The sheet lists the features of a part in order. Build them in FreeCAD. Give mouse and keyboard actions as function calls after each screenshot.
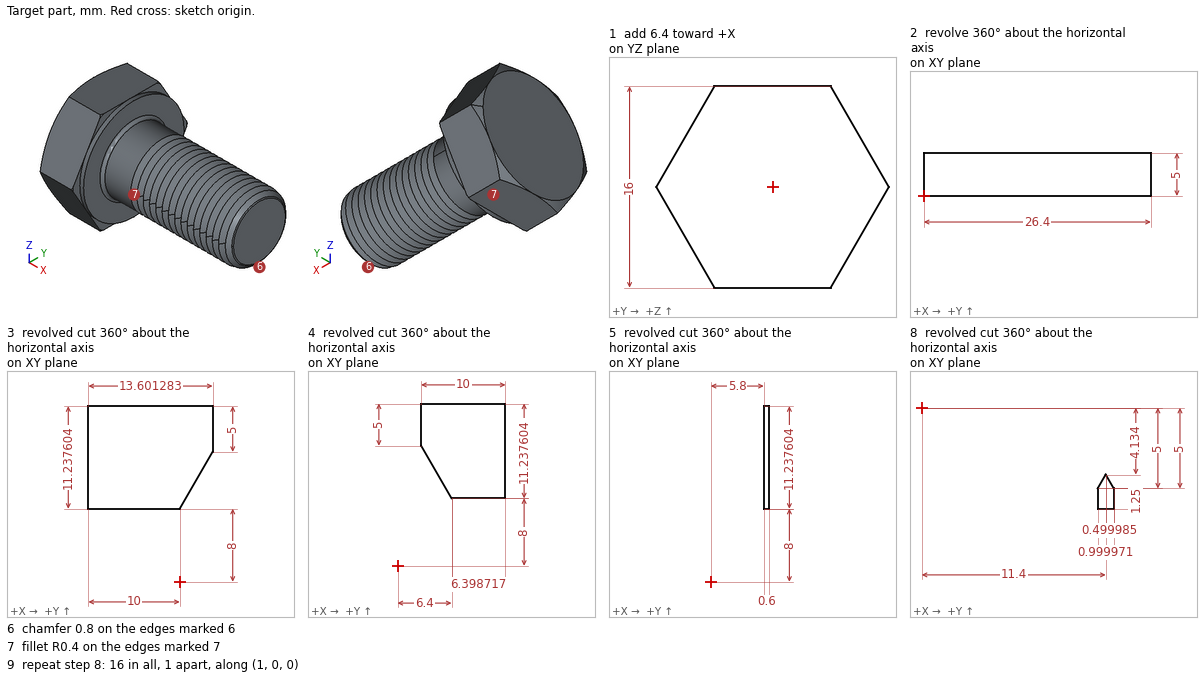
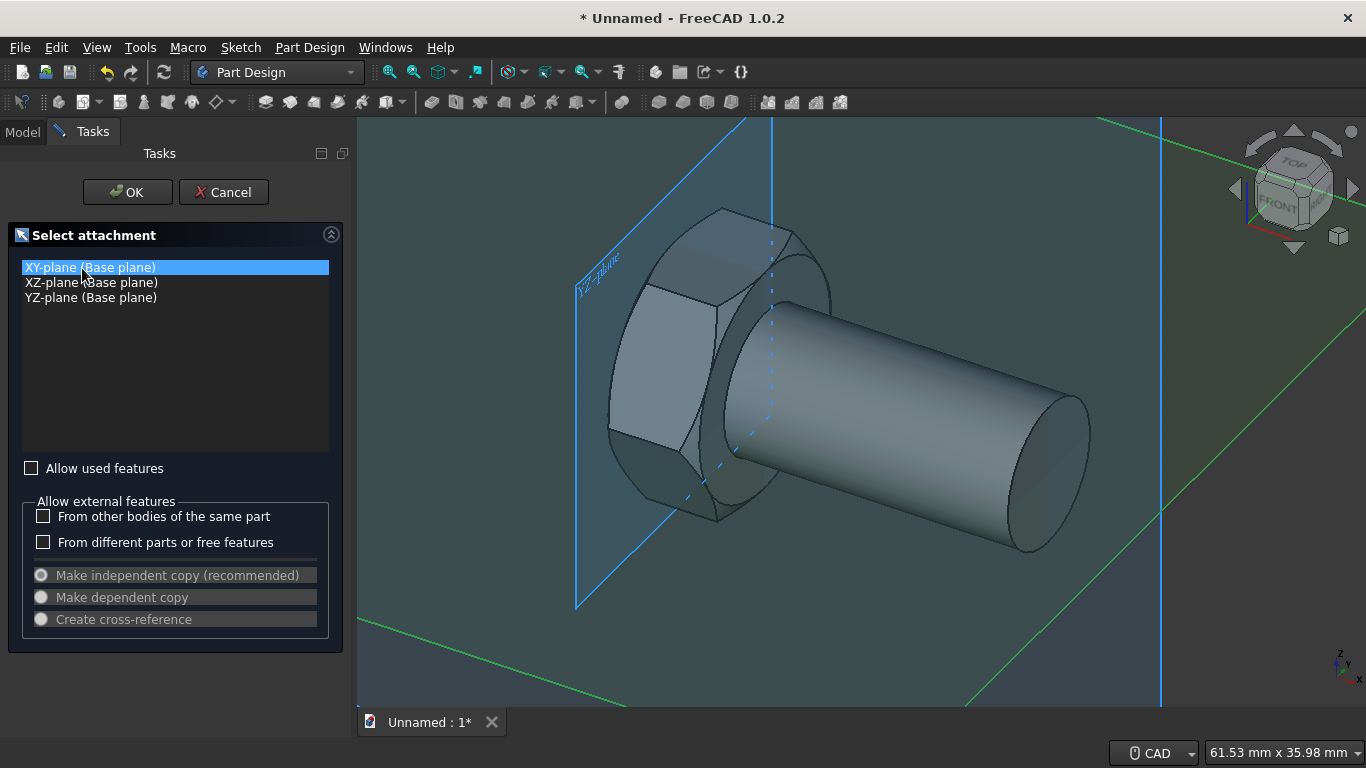
click(128, 192)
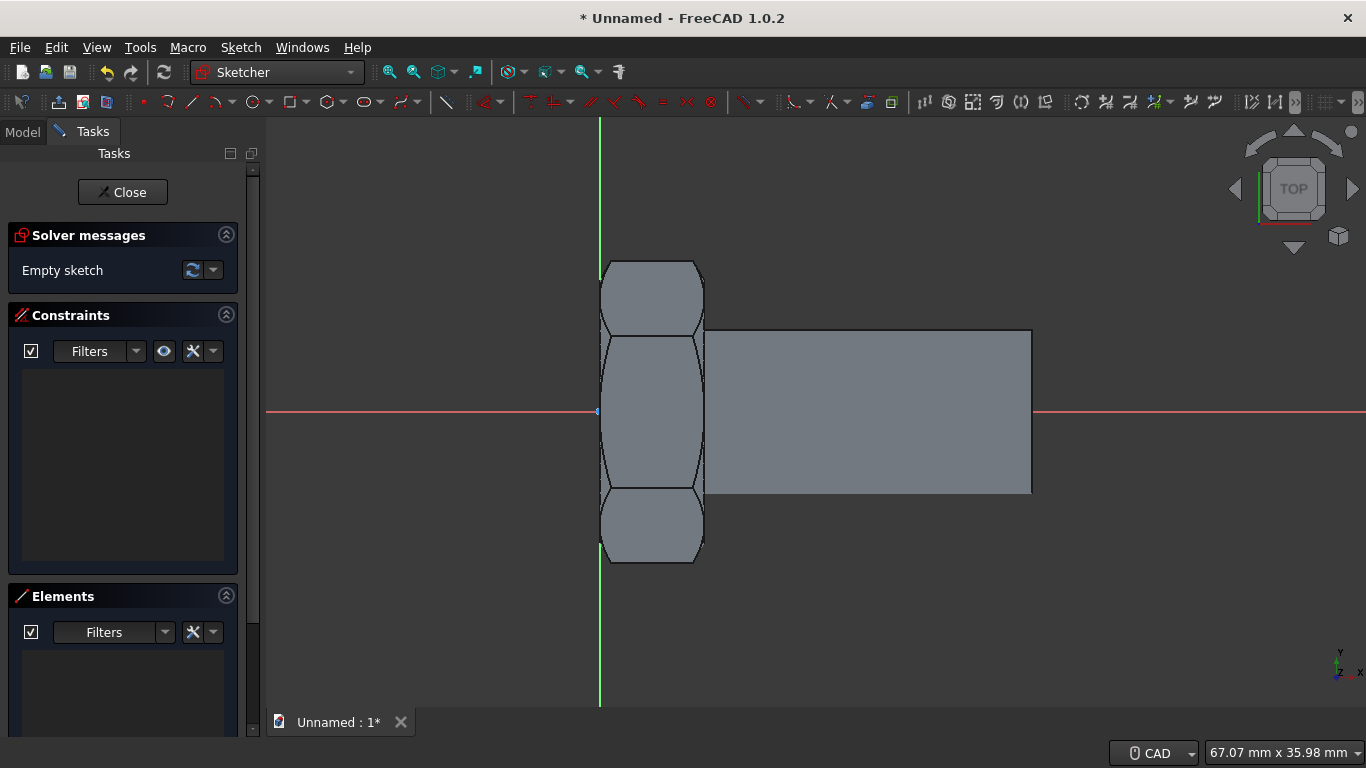
click(108, 102)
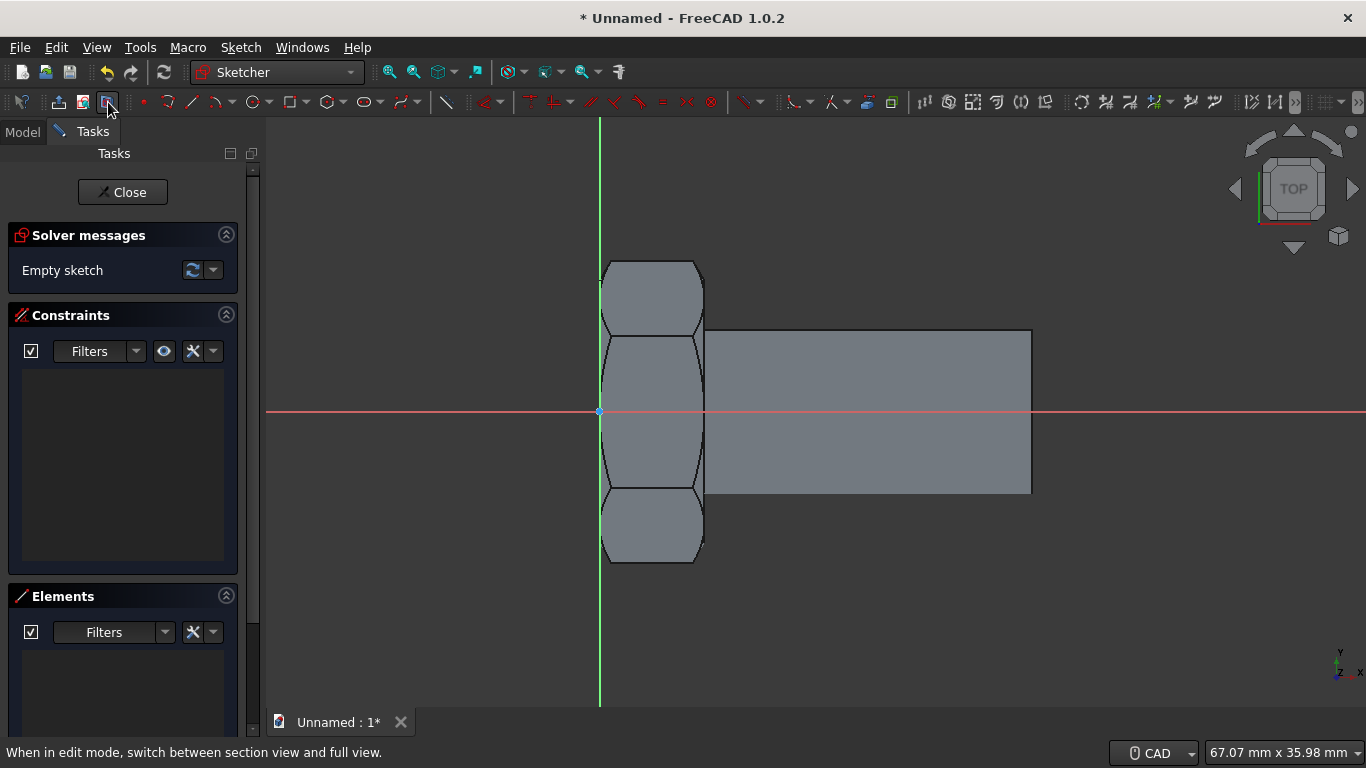
scroll(1179, 679, down, 1)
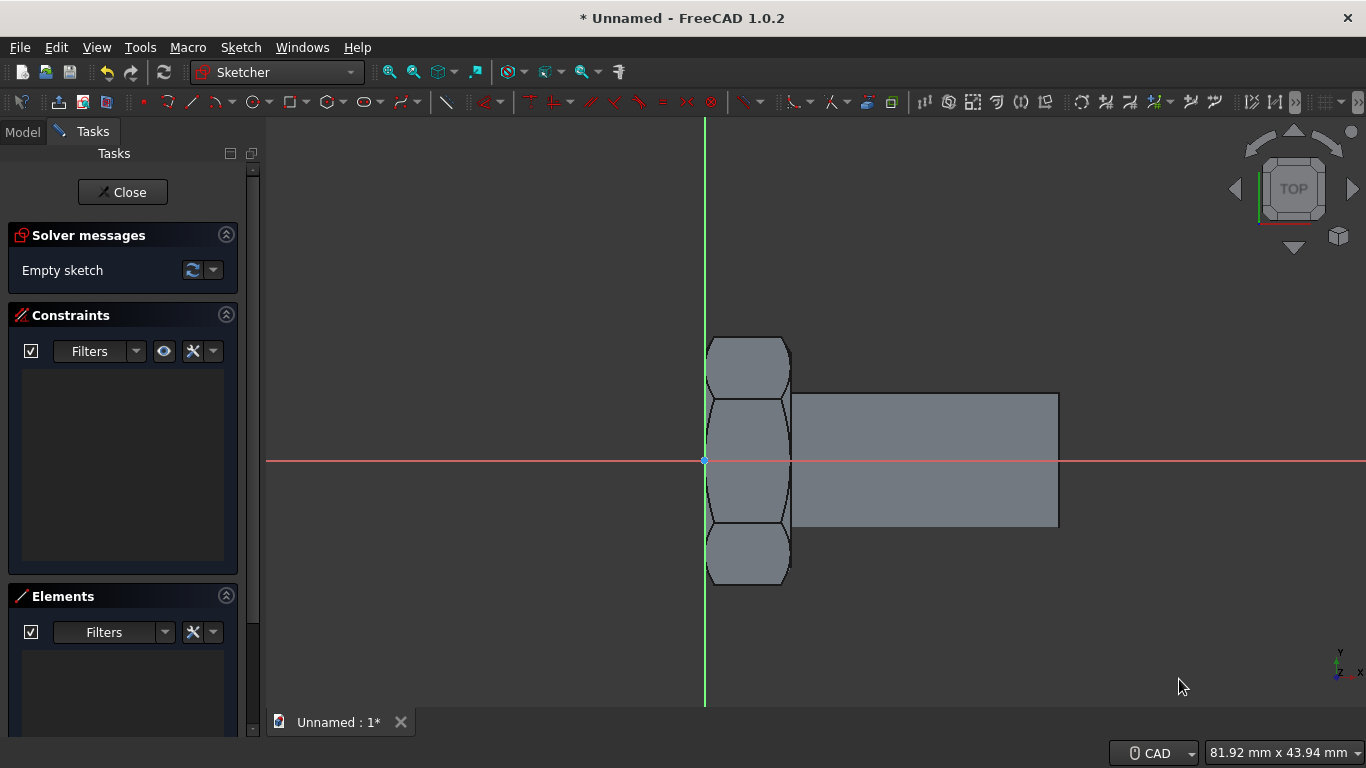
scroll(748, 168, up, 2)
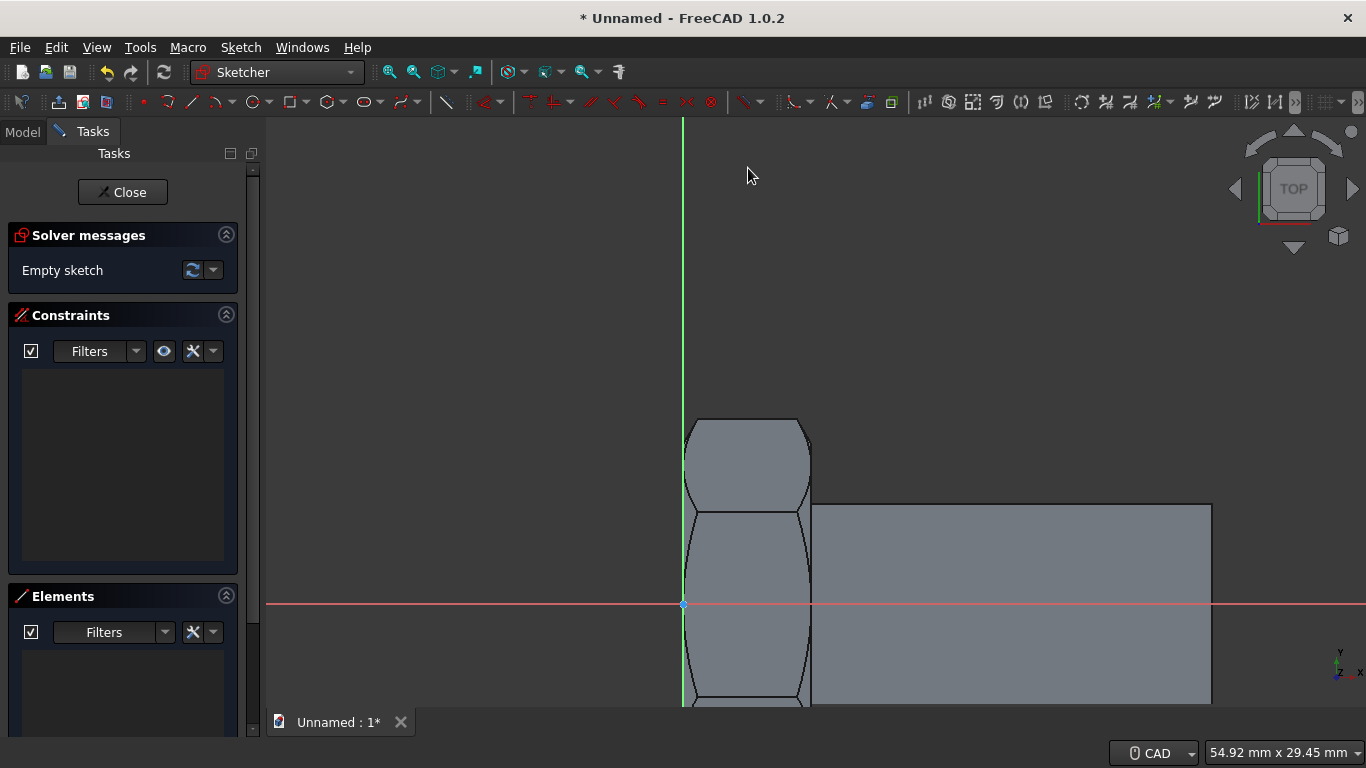
key(g)
key(r)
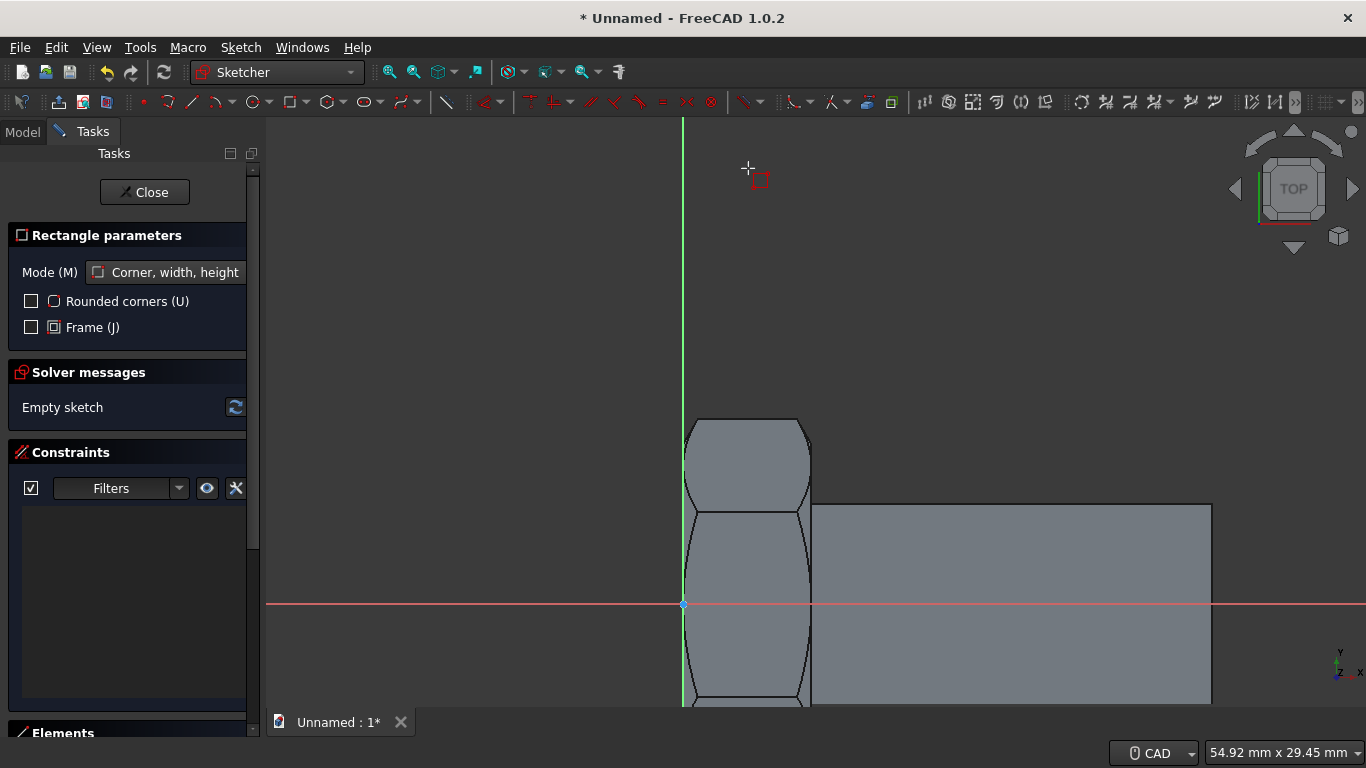
scroll(799, 219, up, 2)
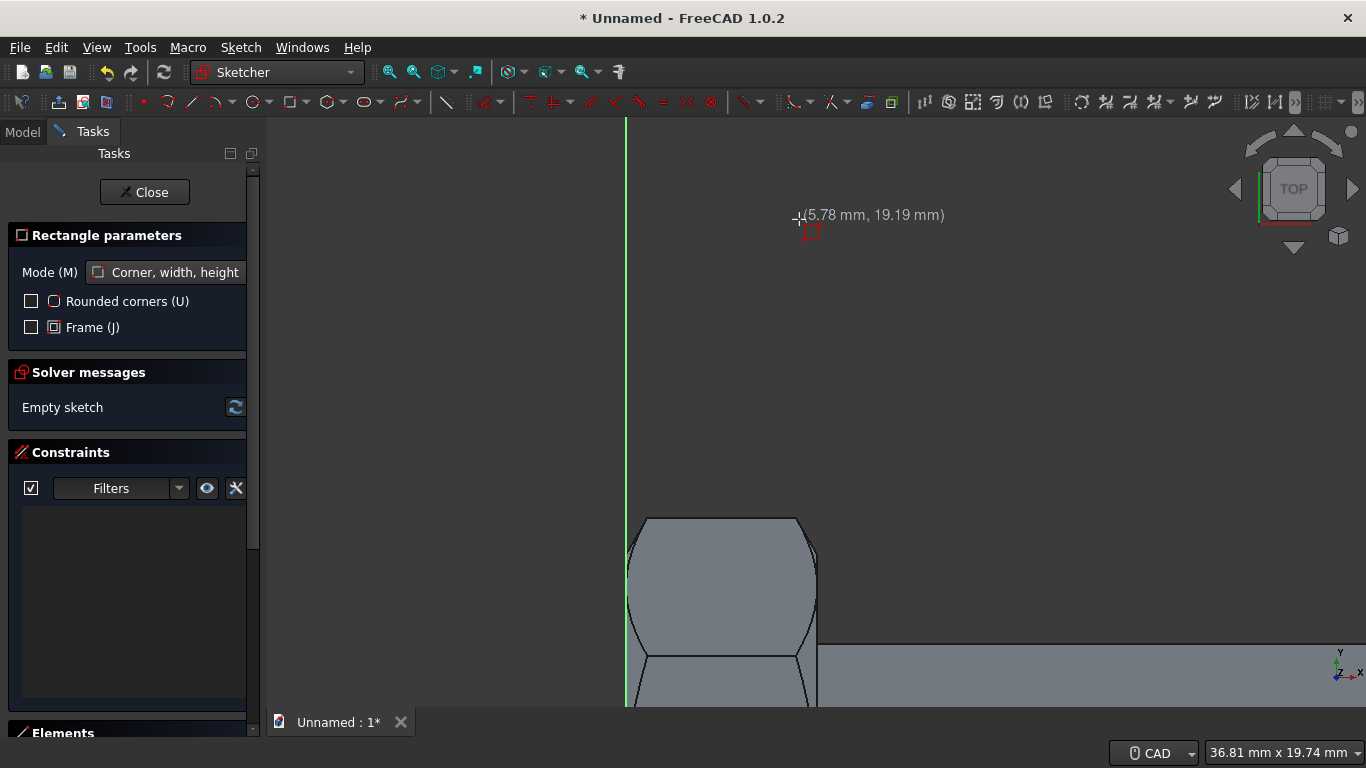
click(799, 219)
click(817, 555)
key(Escape)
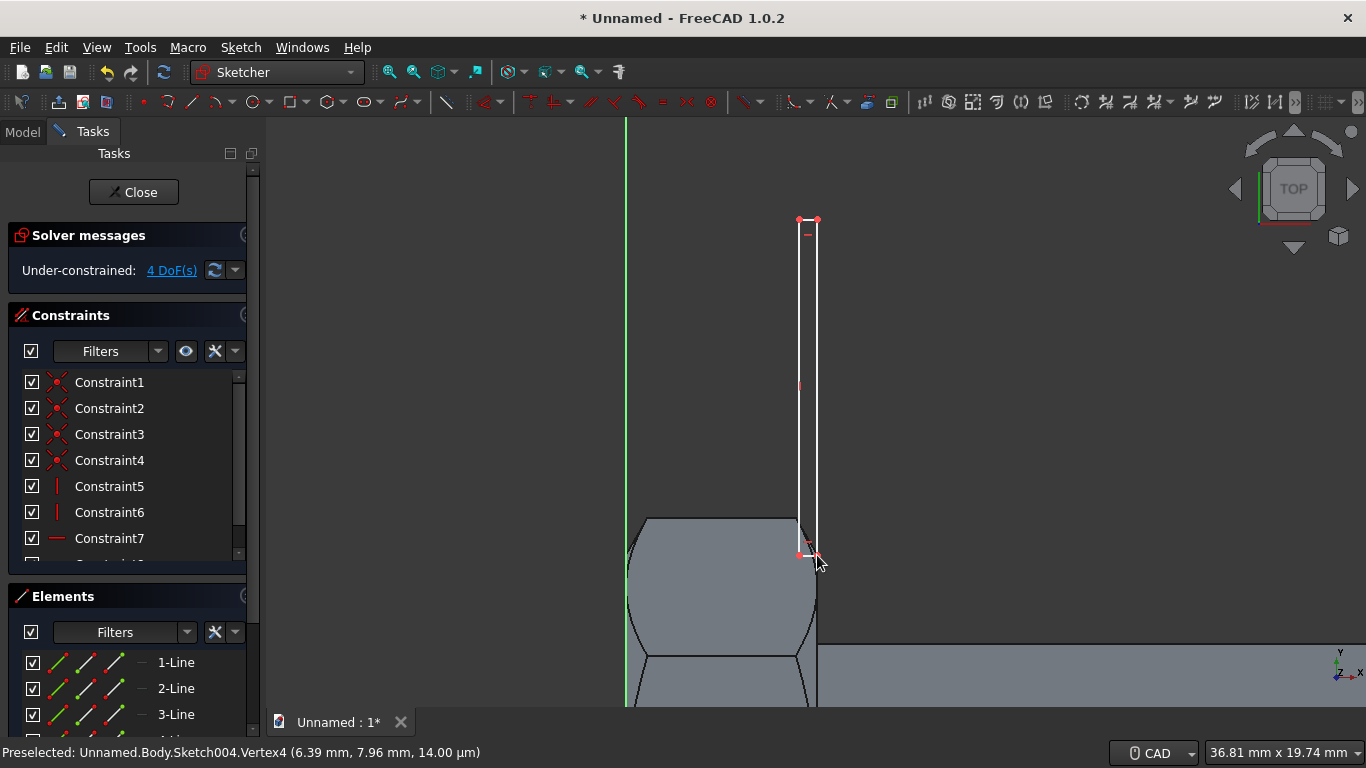
click(484, 102)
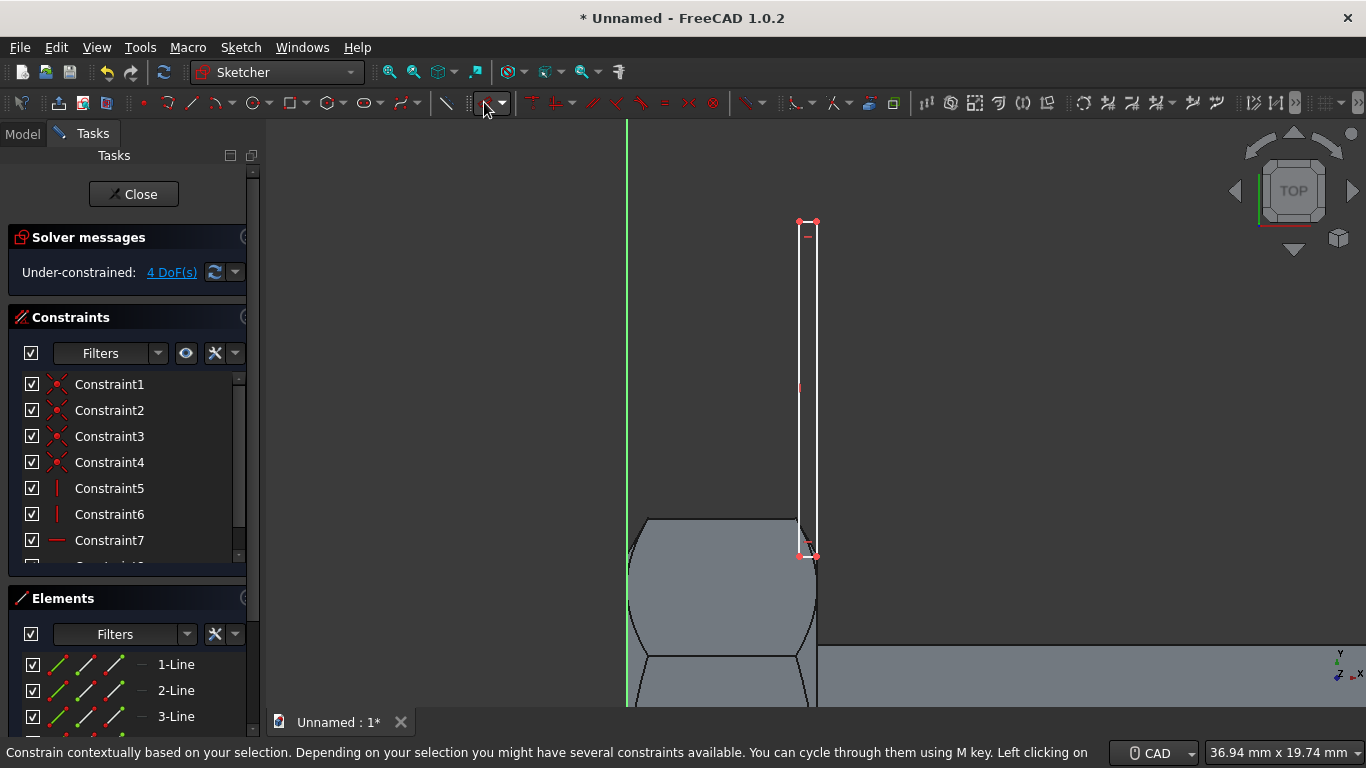
click(799, 557)
click(593, 618)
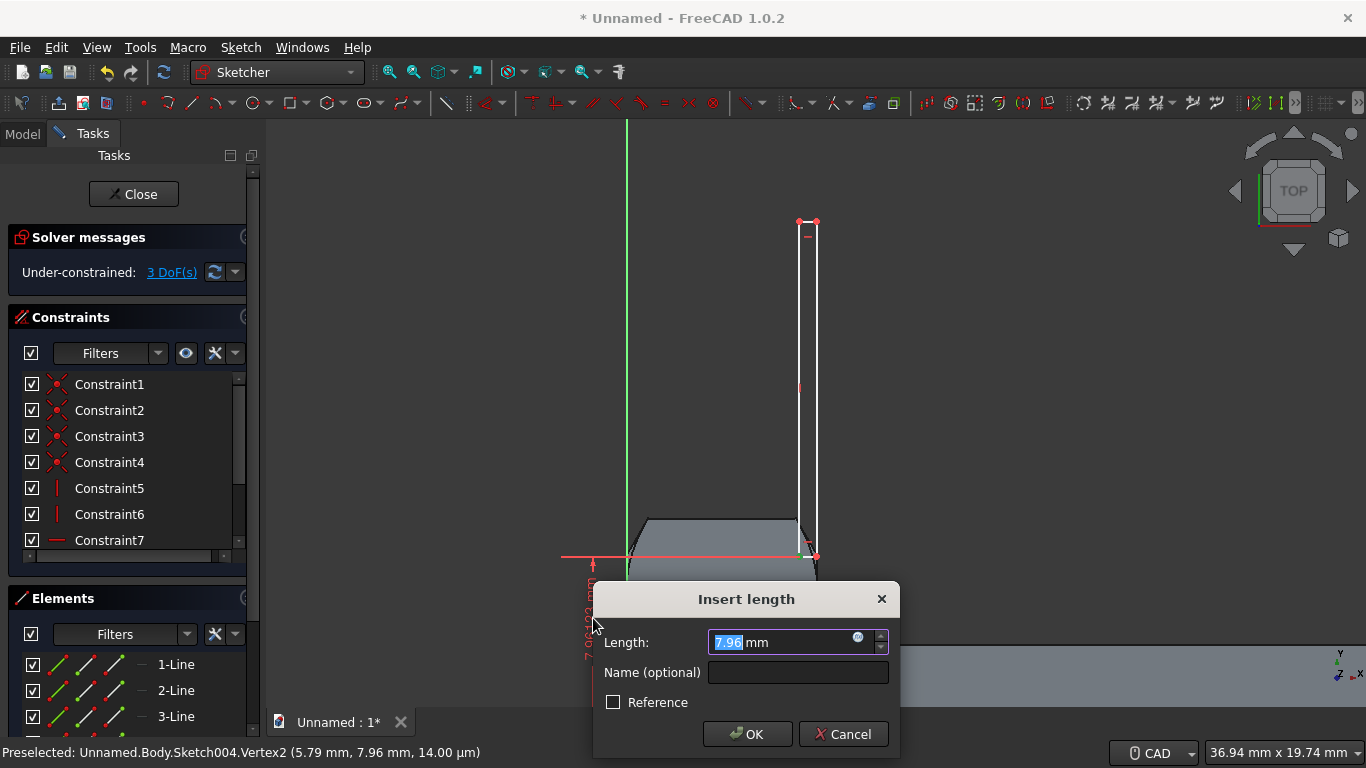
text(8)
key(Return)